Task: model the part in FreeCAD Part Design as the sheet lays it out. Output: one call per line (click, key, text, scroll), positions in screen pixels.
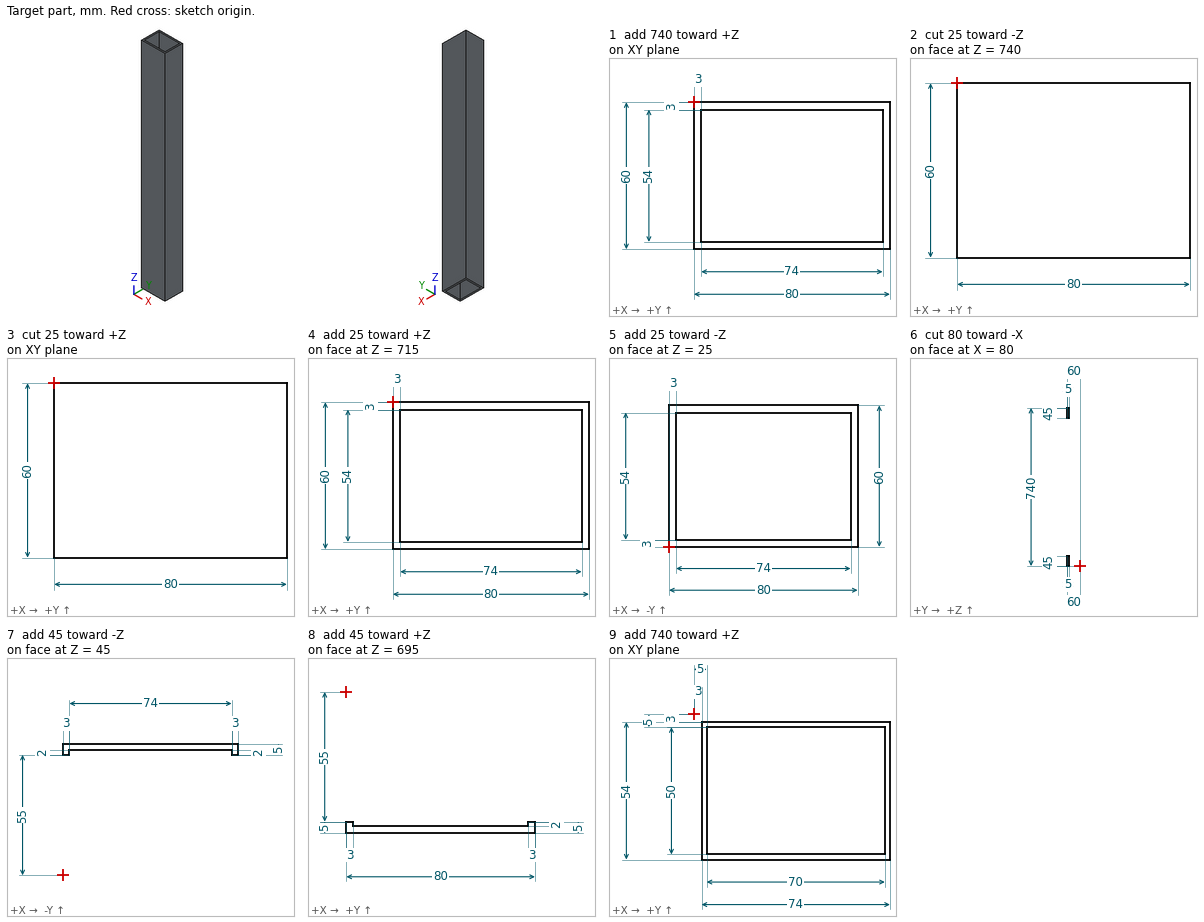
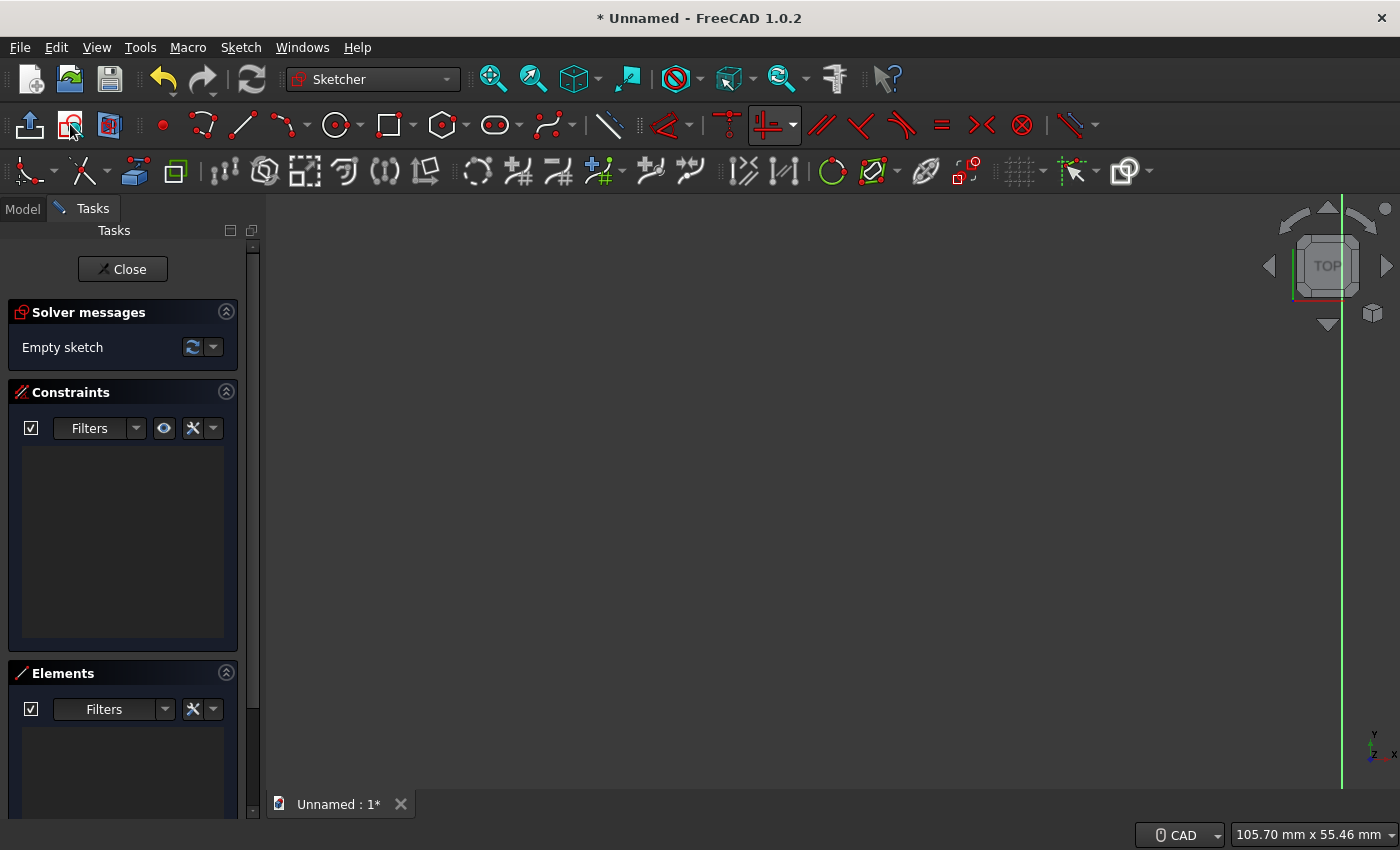
scroll(330, 222, down, 6)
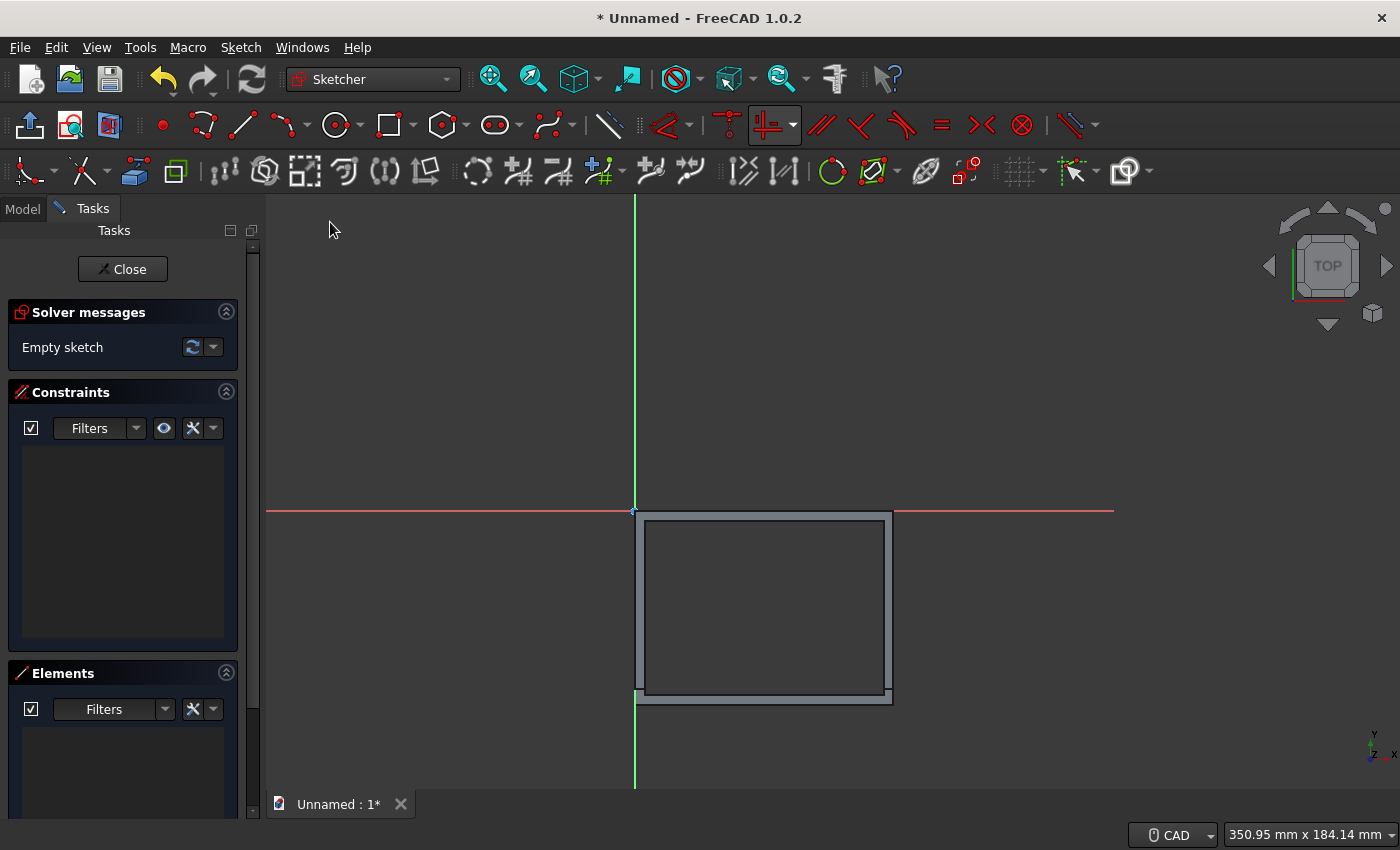
scroll(764, 750, up, 3)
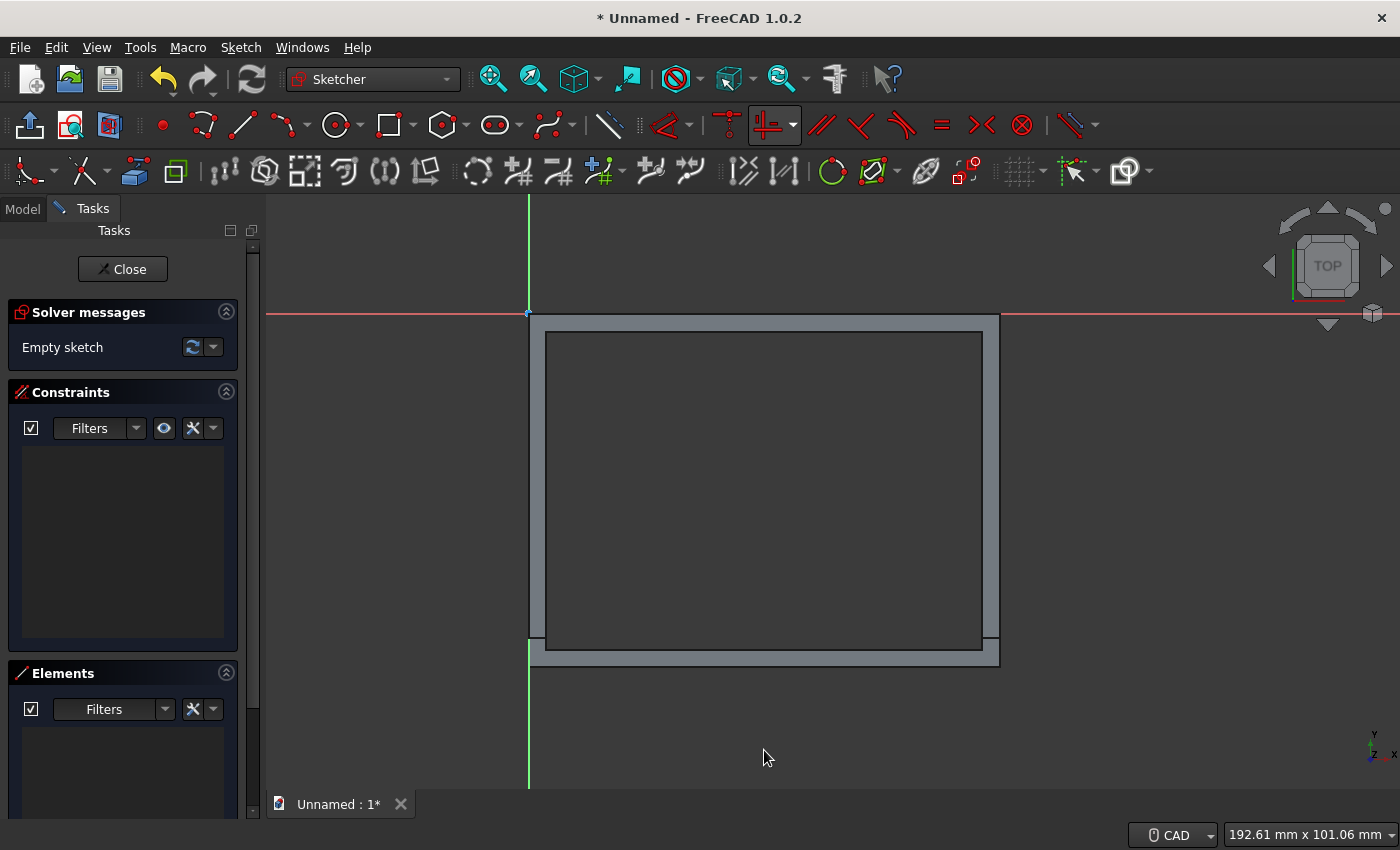
key(g)
key(m)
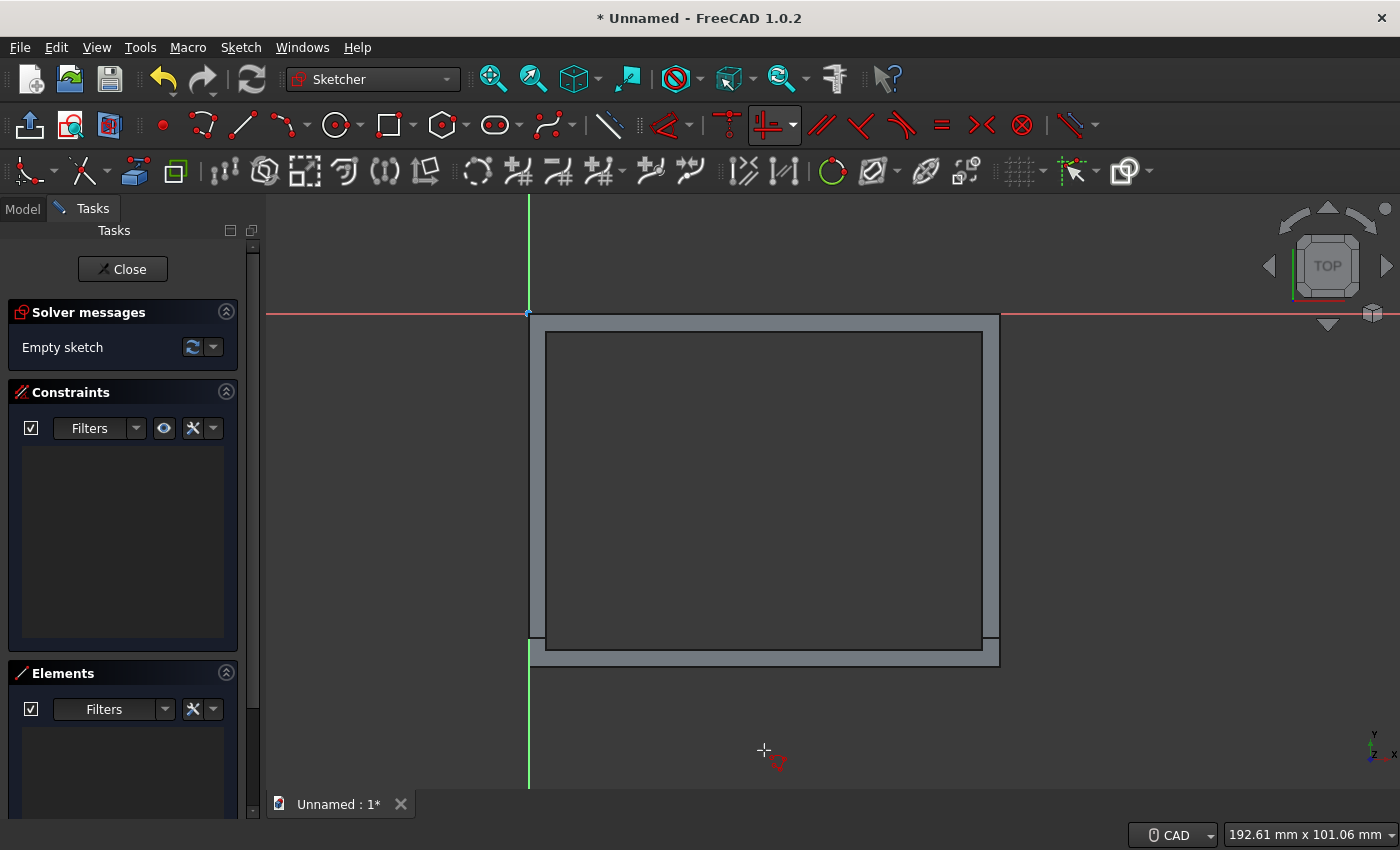
click(529, 638)
click(538, 667)
click(1000, 667)
click(1000, 638)
click(982, 638)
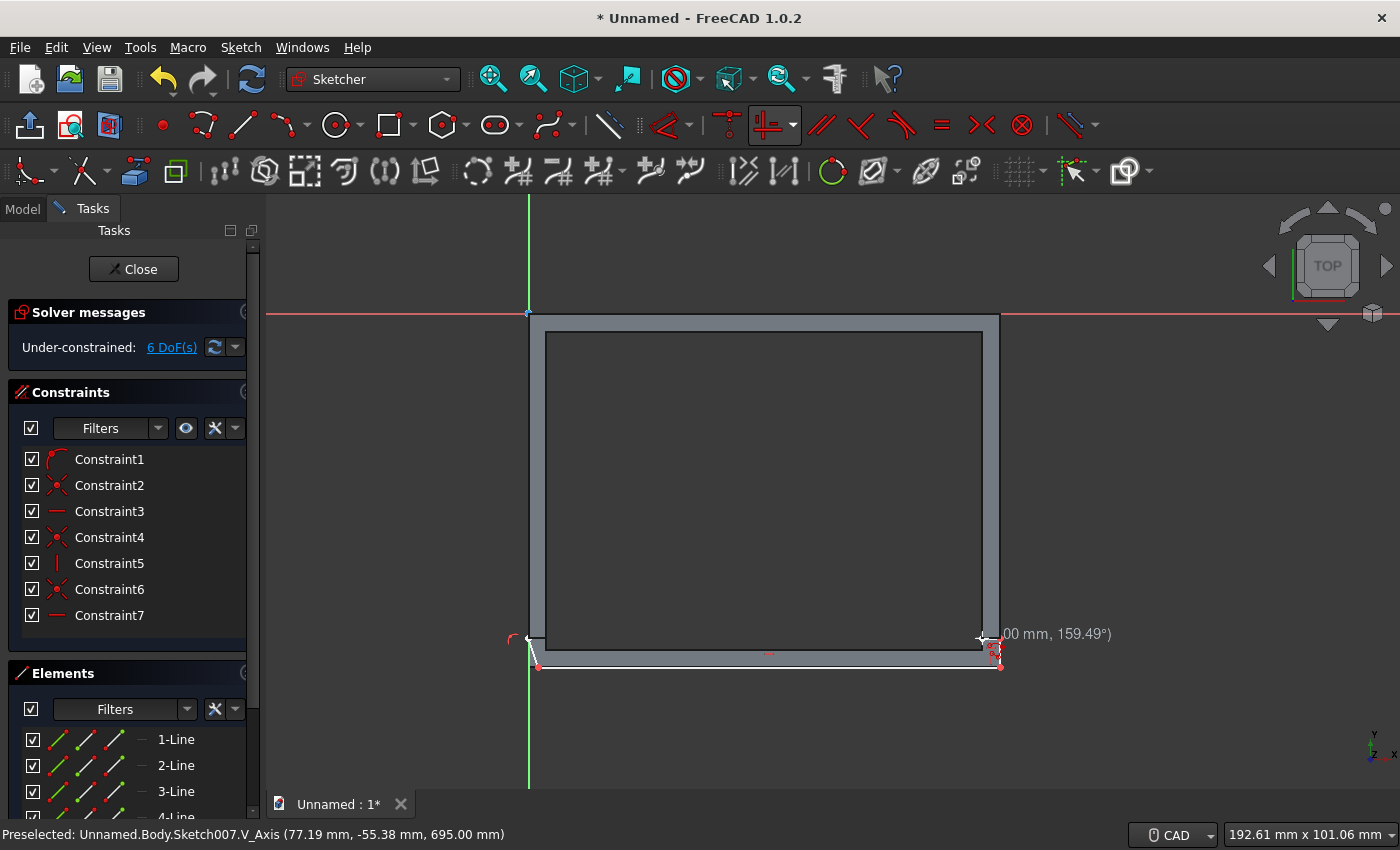
scroll(982, 650, up, 2)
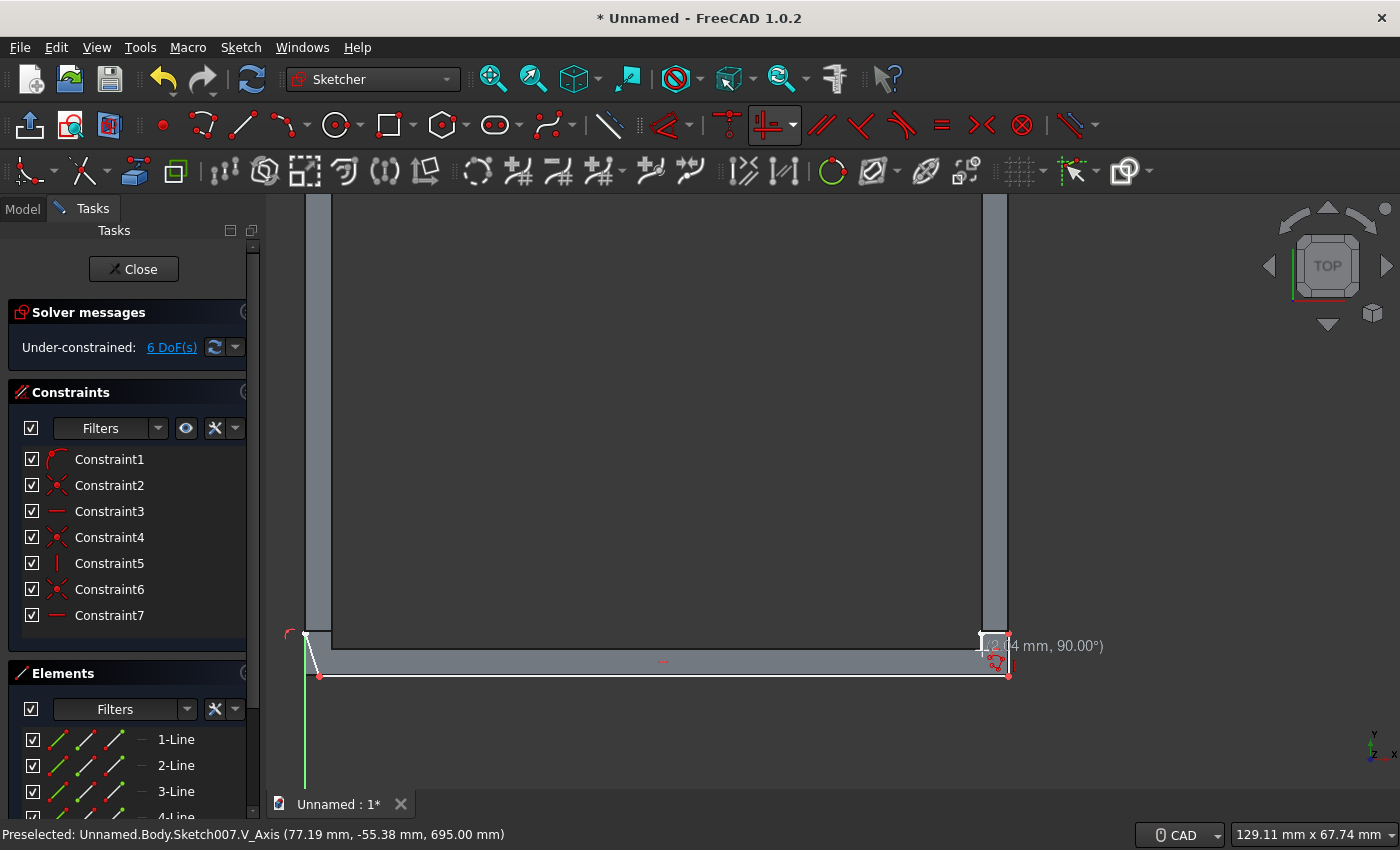
click(982, 649)
click(332, 649)
click(332, 631)
click(305, 633)
key(Escape)
key(Escape)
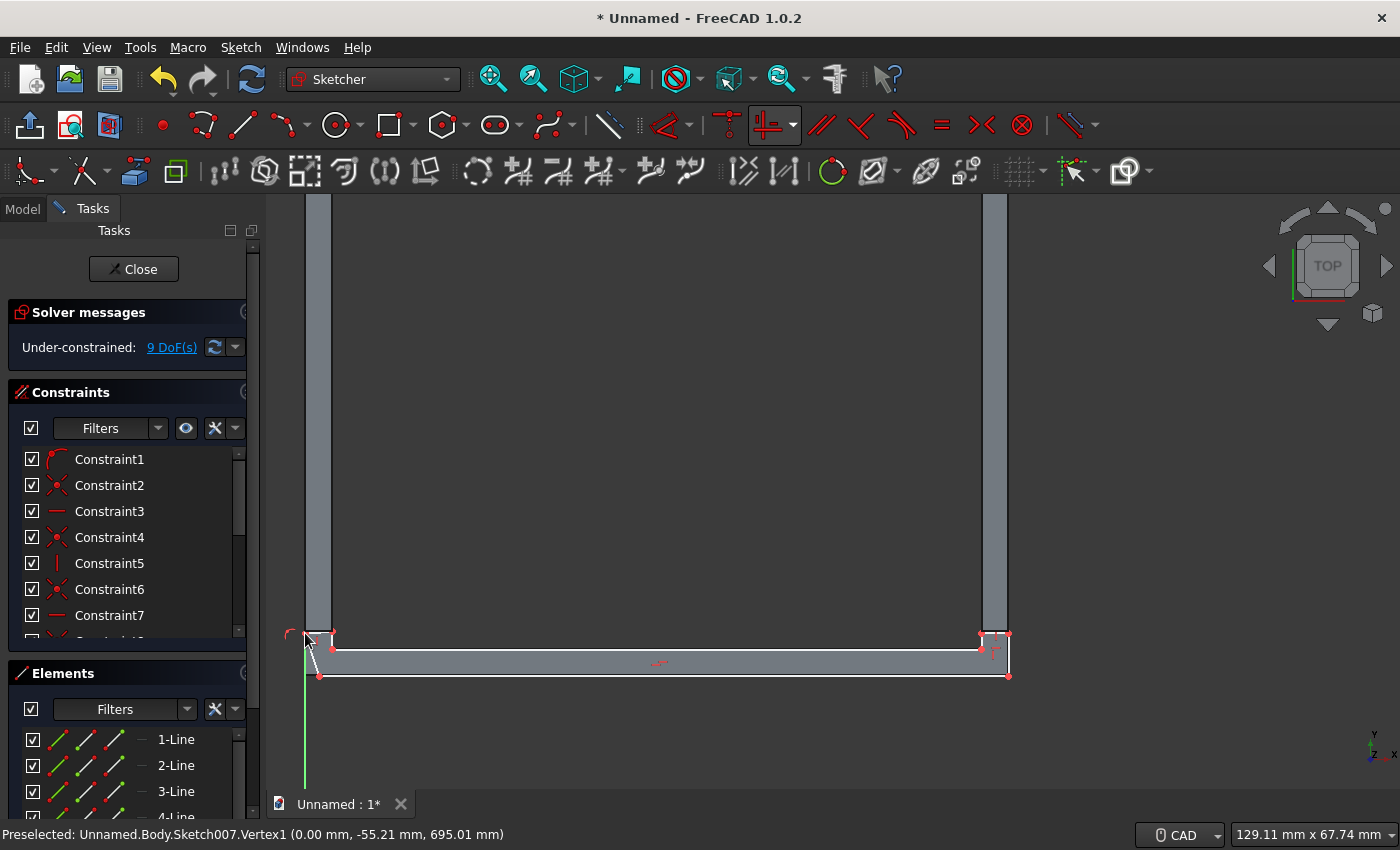
scroll(315, 663, up, 2)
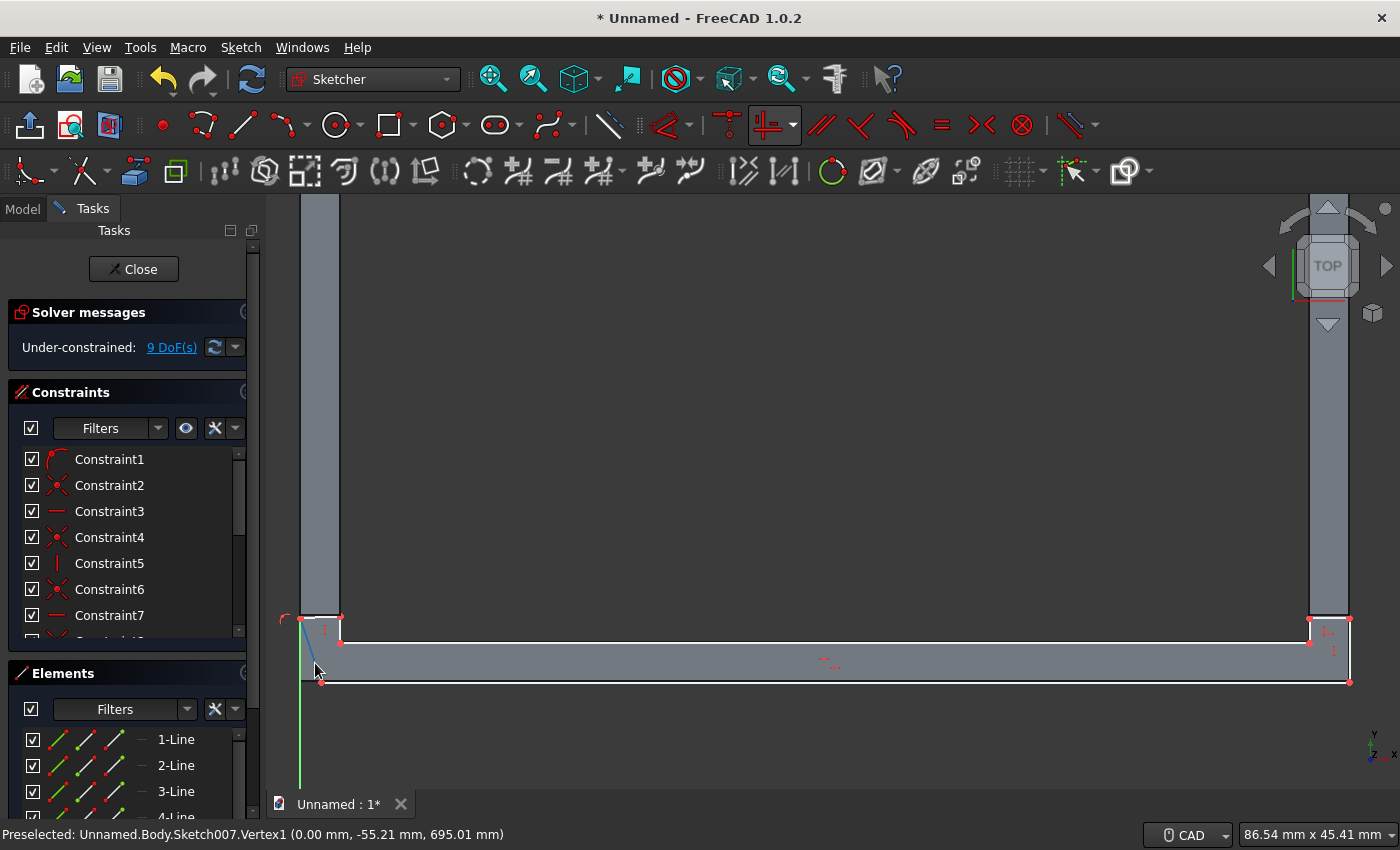
click(315, 663)